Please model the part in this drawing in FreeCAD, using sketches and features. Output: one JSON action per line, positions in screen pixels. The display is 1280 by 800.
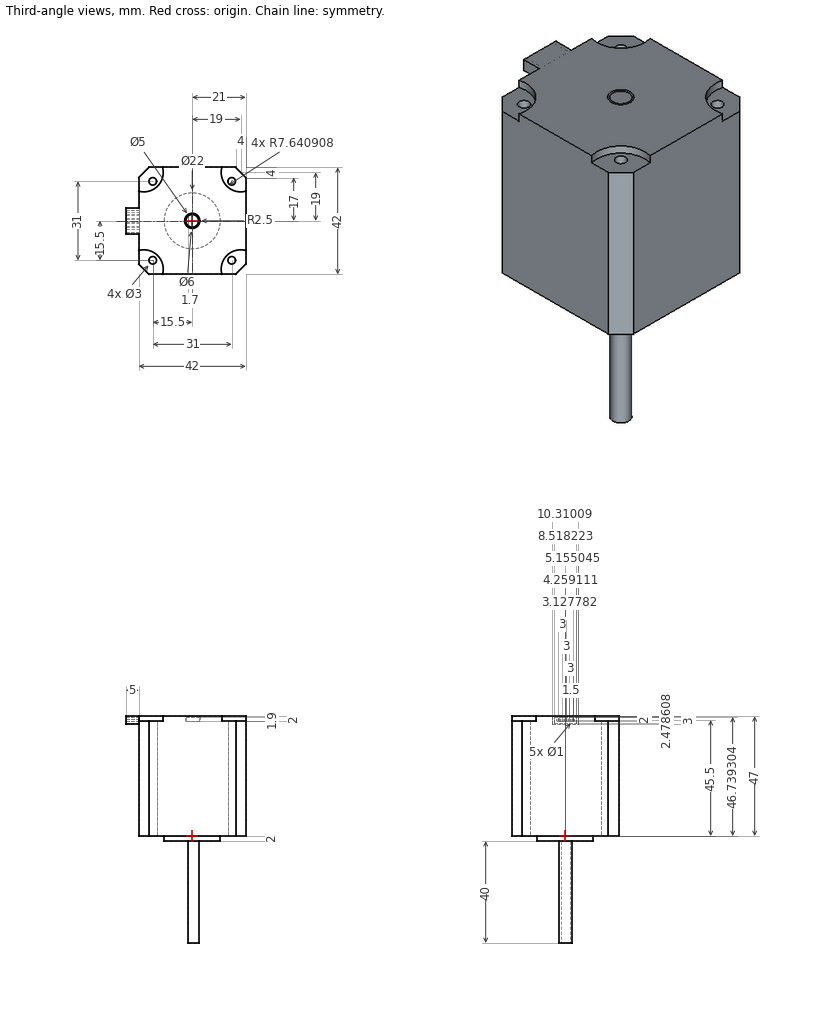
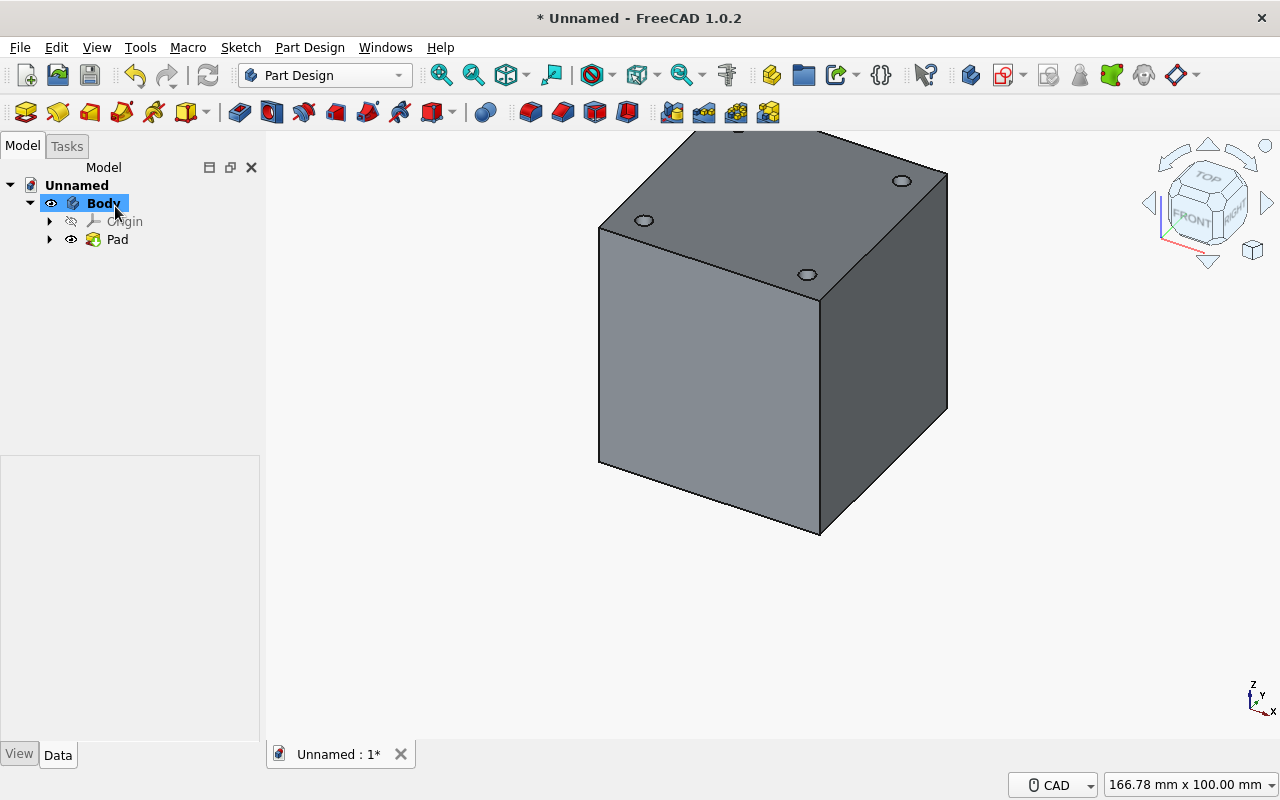
{"action": "left_click", "coordinate": [442, 76]}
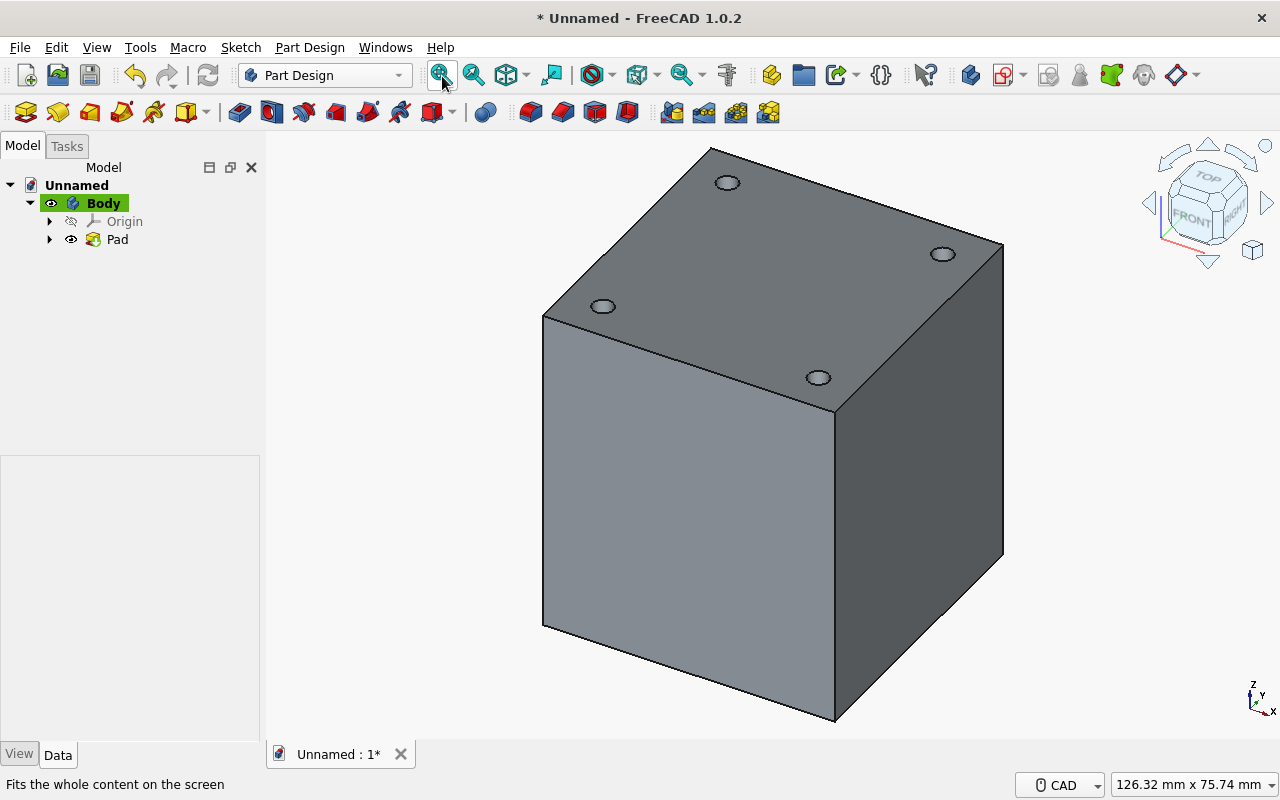
{"action": "key", "text": "5"}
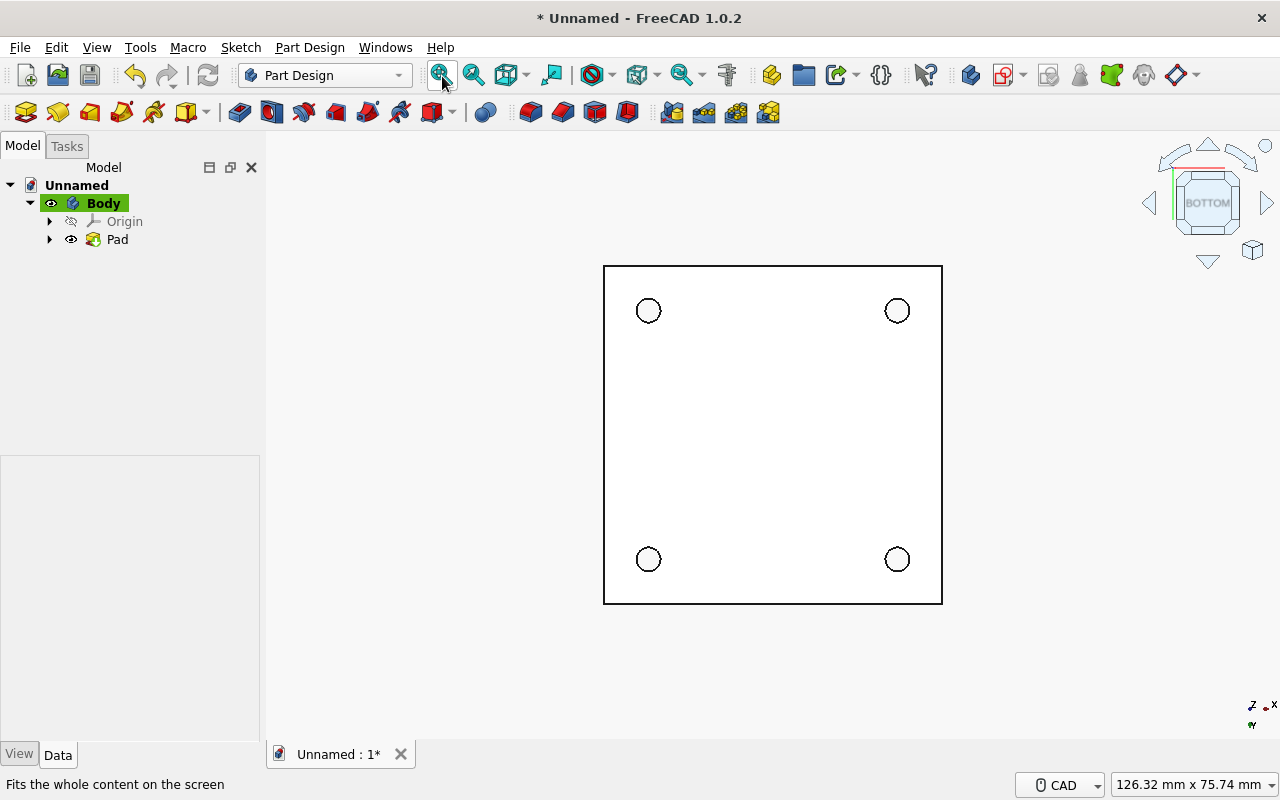
{"action": "left_click", "coordinate": [773, 434]}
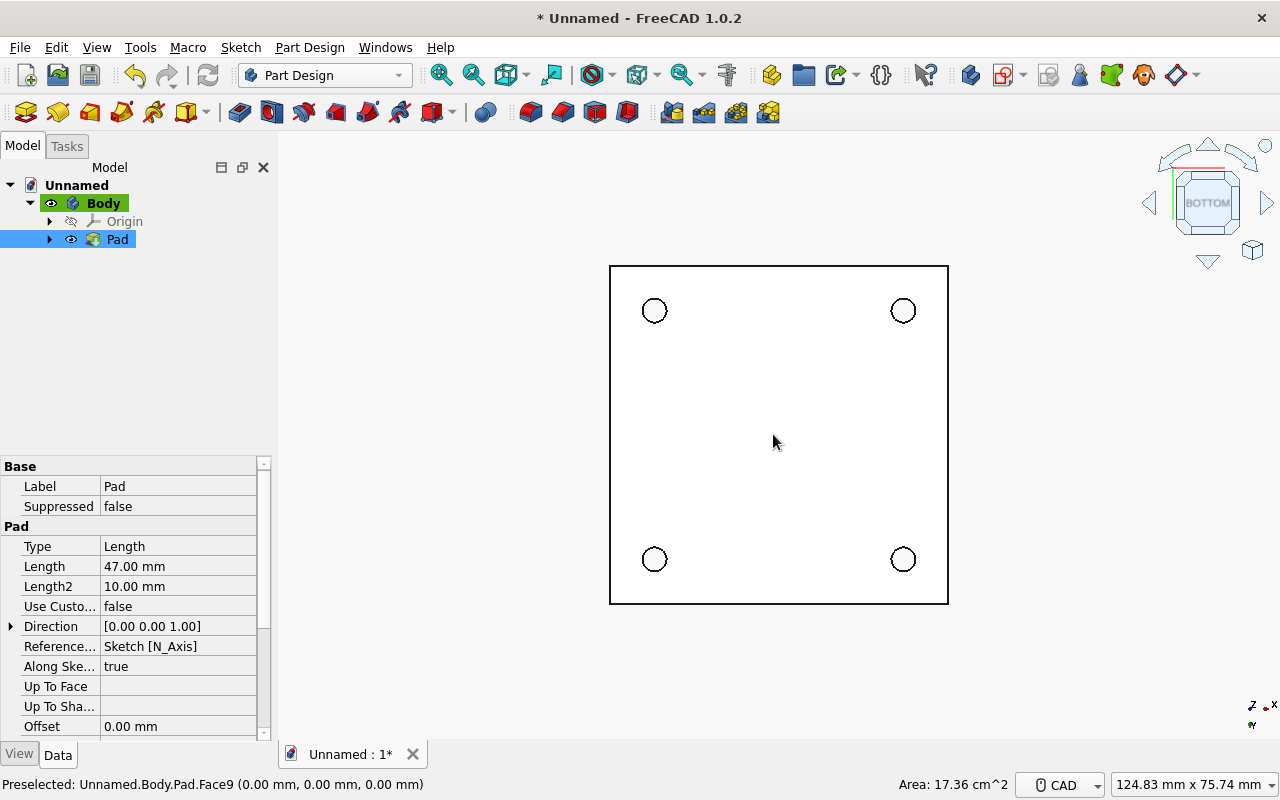
{"action": "left_click", "coordinate": [1004, 76]}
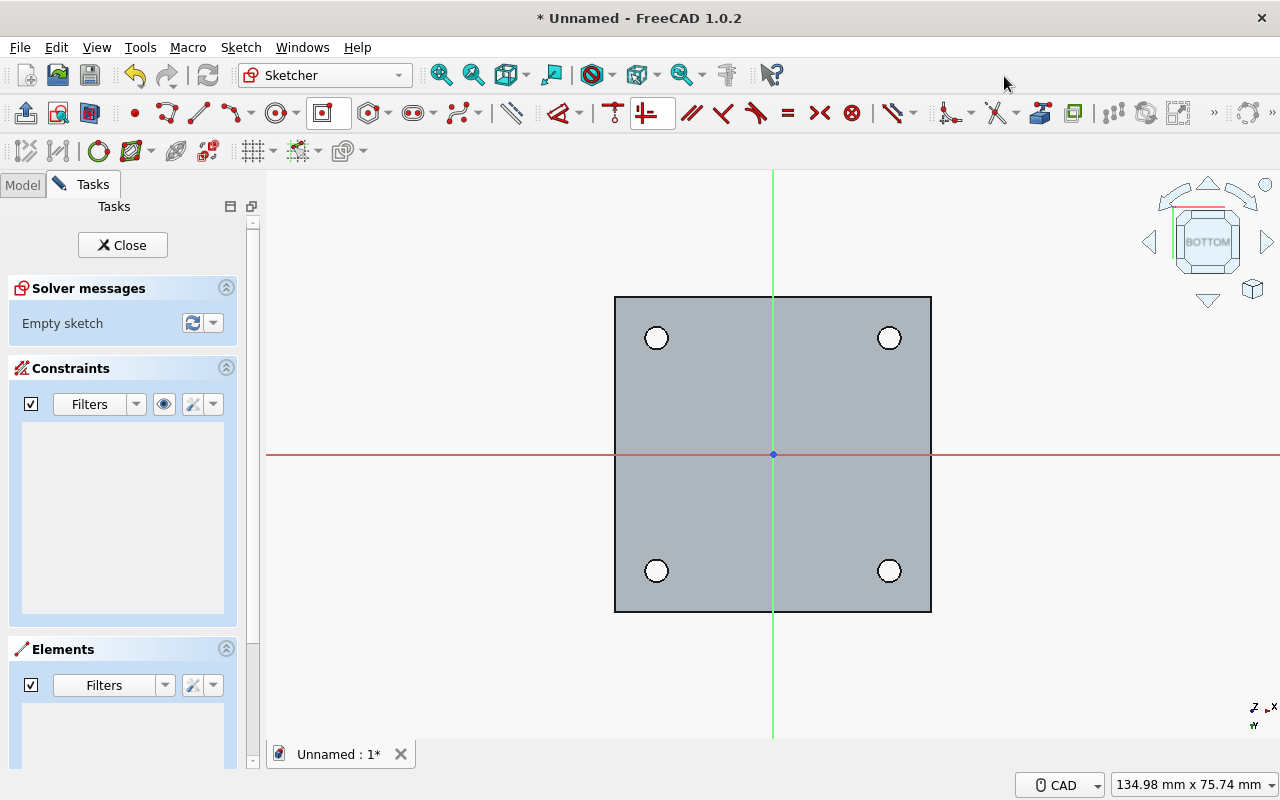
{"action": "left_click", "coordinate": [168, 114]}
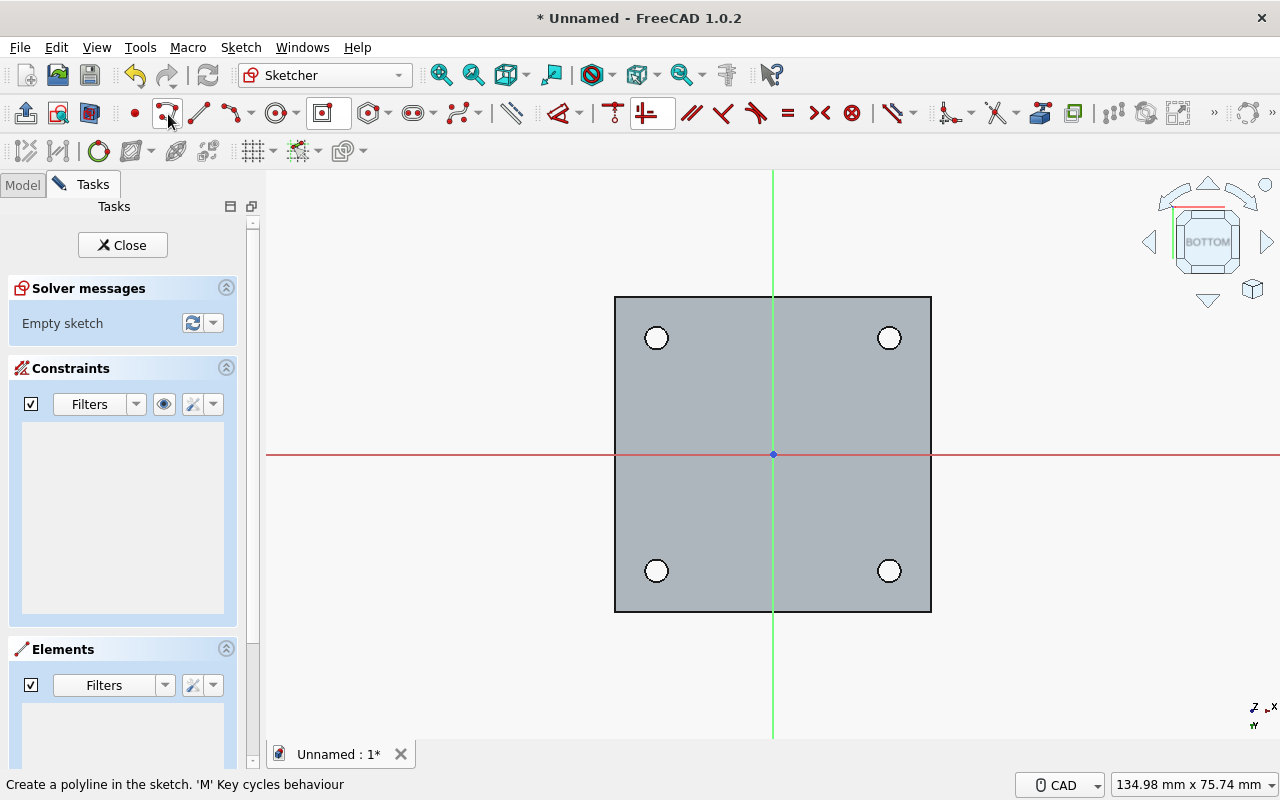
{"action": "left_click", "coordinate": [931, 582]}
{"action": "left_click", "coordinate": [901, 612]}
{"action": "left_click", "coordinate": [931, 612]}
{"action": "left_click", "coordinate": [931, 583]}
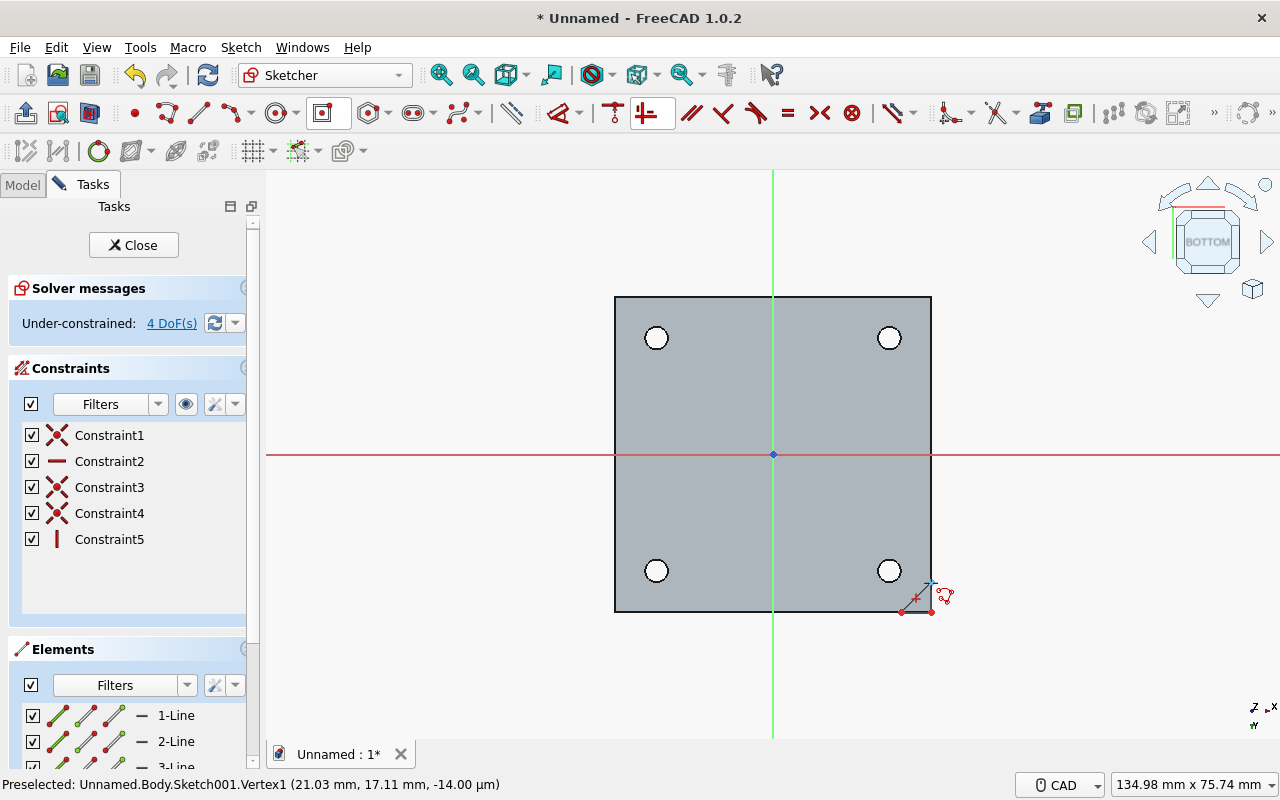
{"action": "left_click", "coordinate": [645, 612]}
{"action": "left_click", "coordinate": [615, 582]}
{"action": "left_click", "coordinate": [615, 612]}
{"action": "left_click", "coordinate": [645, 613]}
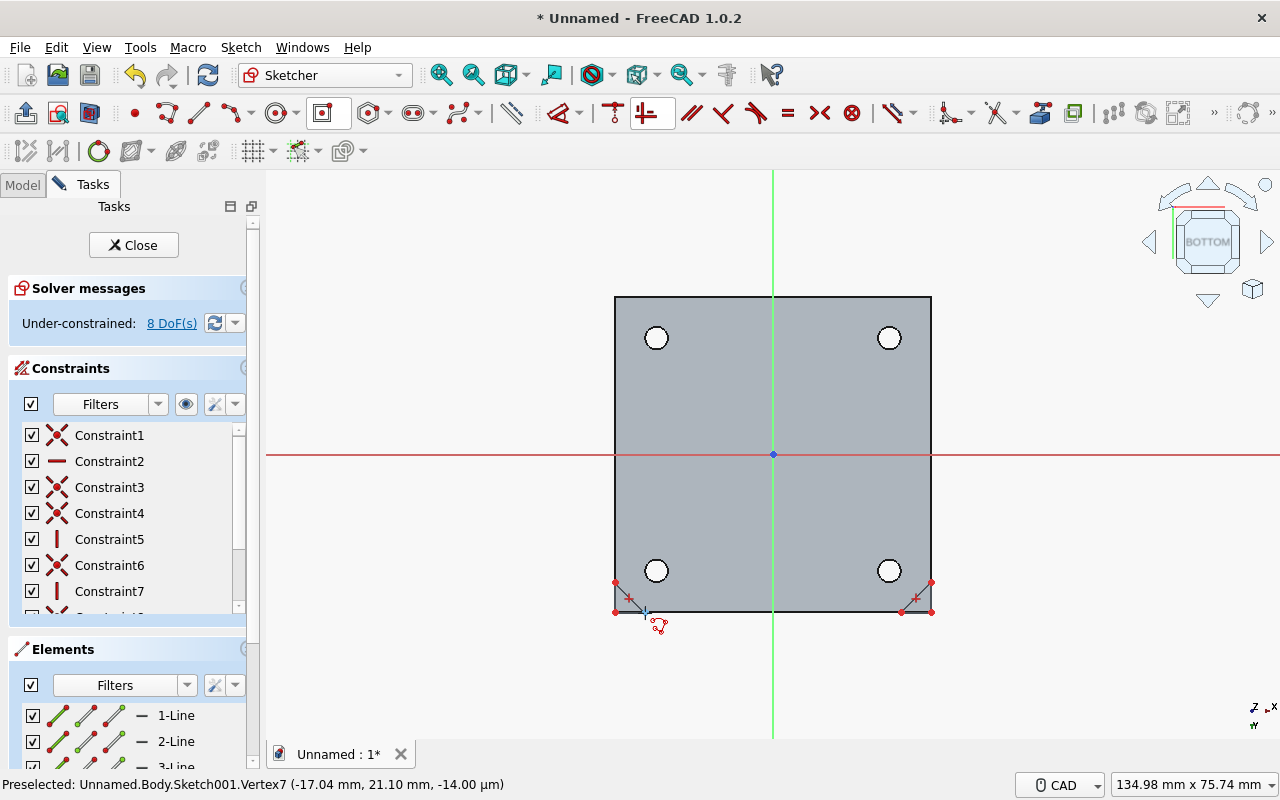
{"action": "left_click", "coordinate": [615, 327]}
{"action": "left_click", "coordinate": [645, 297]}
{"action": "left_click", "coordinate": [615, 297]}
{"action": "left_click", "coordinate": [615, 328]}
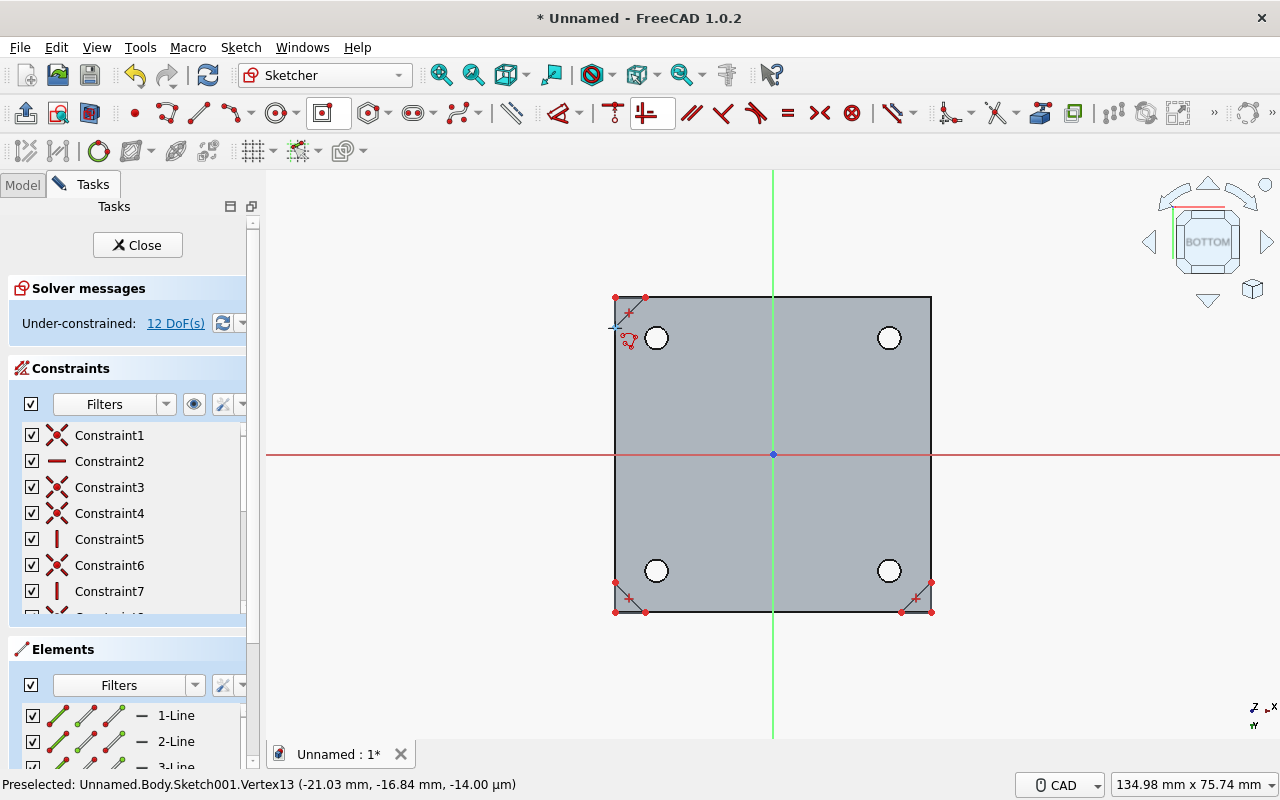
{"action": "left_click", "coordinate": [901, 297]}
{"action": "left_click", "coordinate": [931, 327]}
{"action": "left_click", "coordinate": [931, 297]}
{"action": "left_click", "coordinate": [901, 298]}
{"action": "key", "text": "Escape"}
{"action": "key", "text": "Escape"}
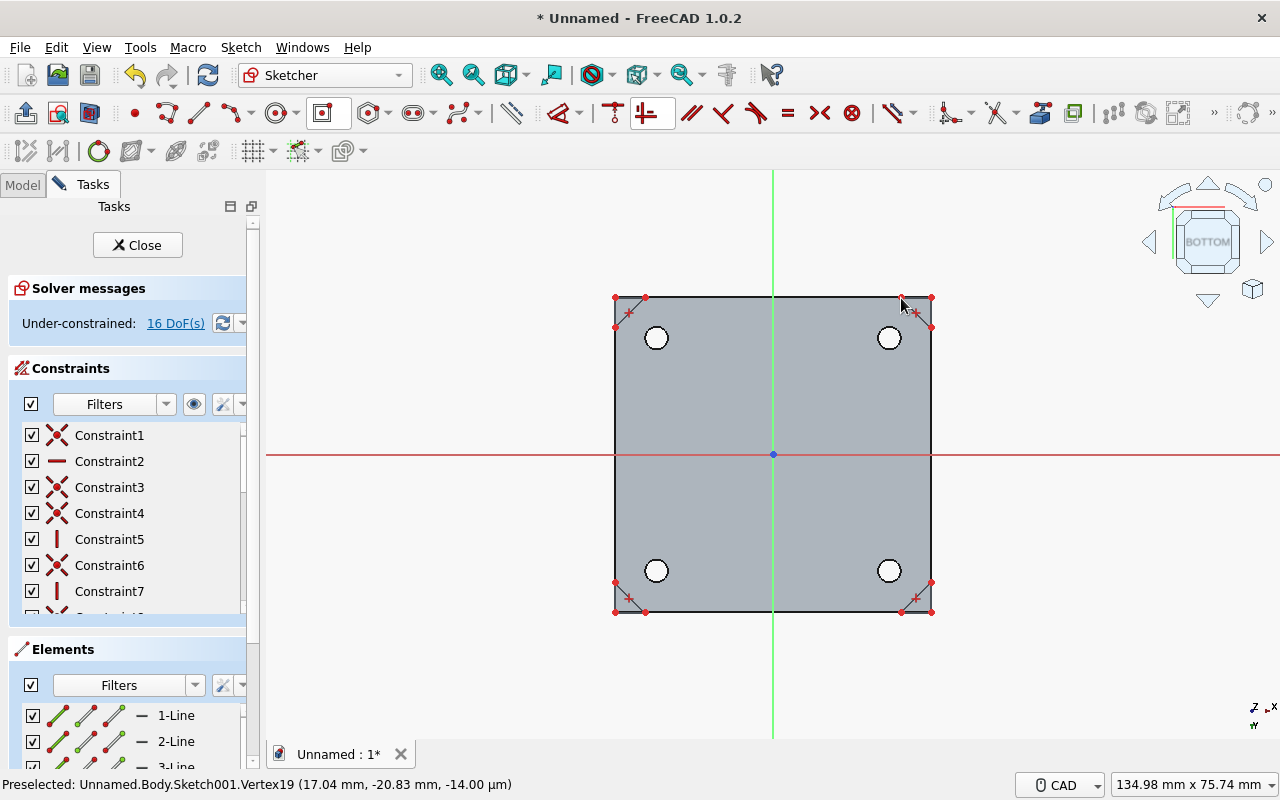
{"action": "left_click", "coordinate": [901, 613]}